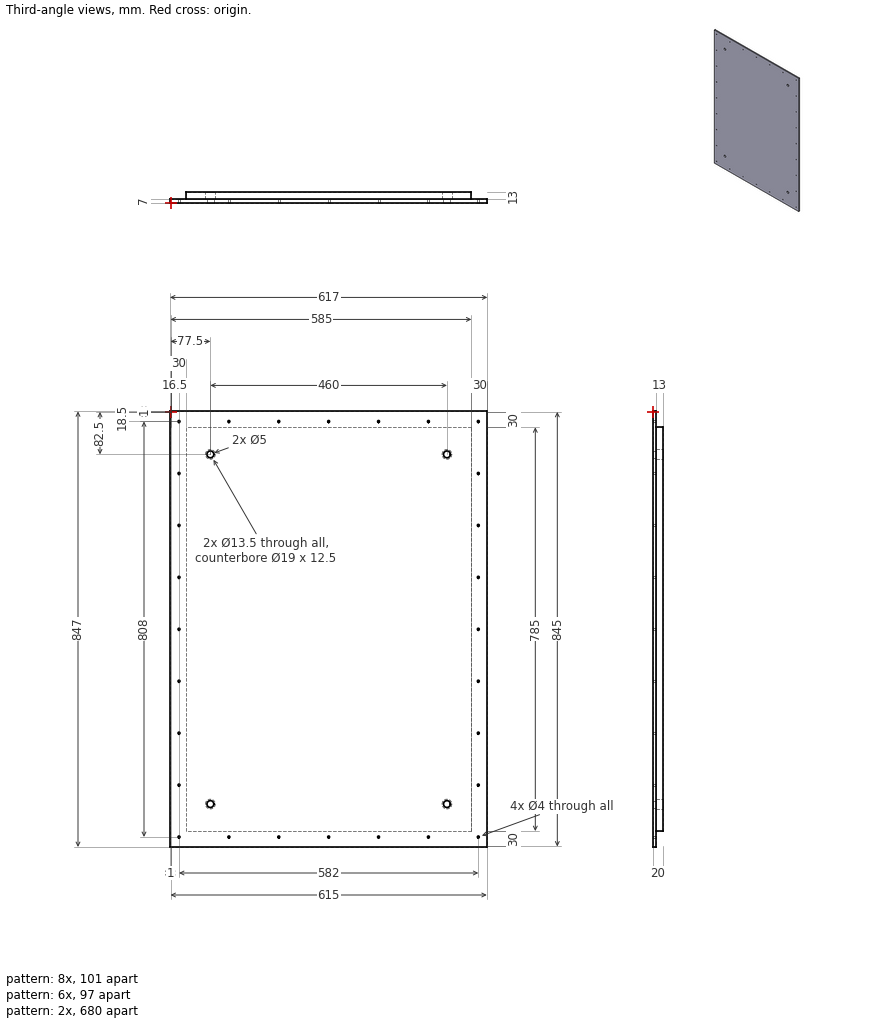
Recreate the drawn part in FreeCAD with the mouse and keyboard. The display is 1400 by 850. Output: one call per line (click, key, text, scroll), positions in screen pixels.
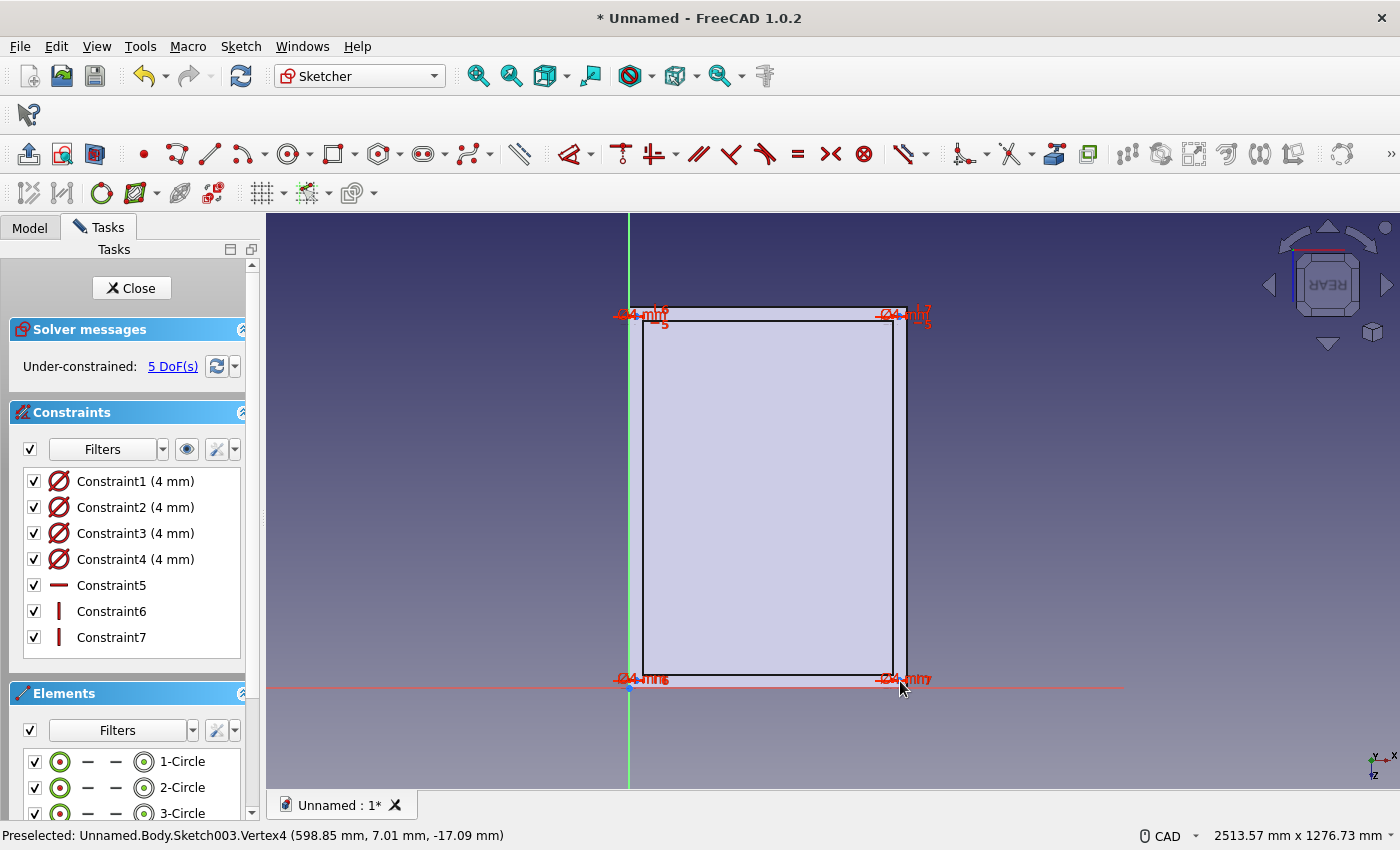
click(637, 681)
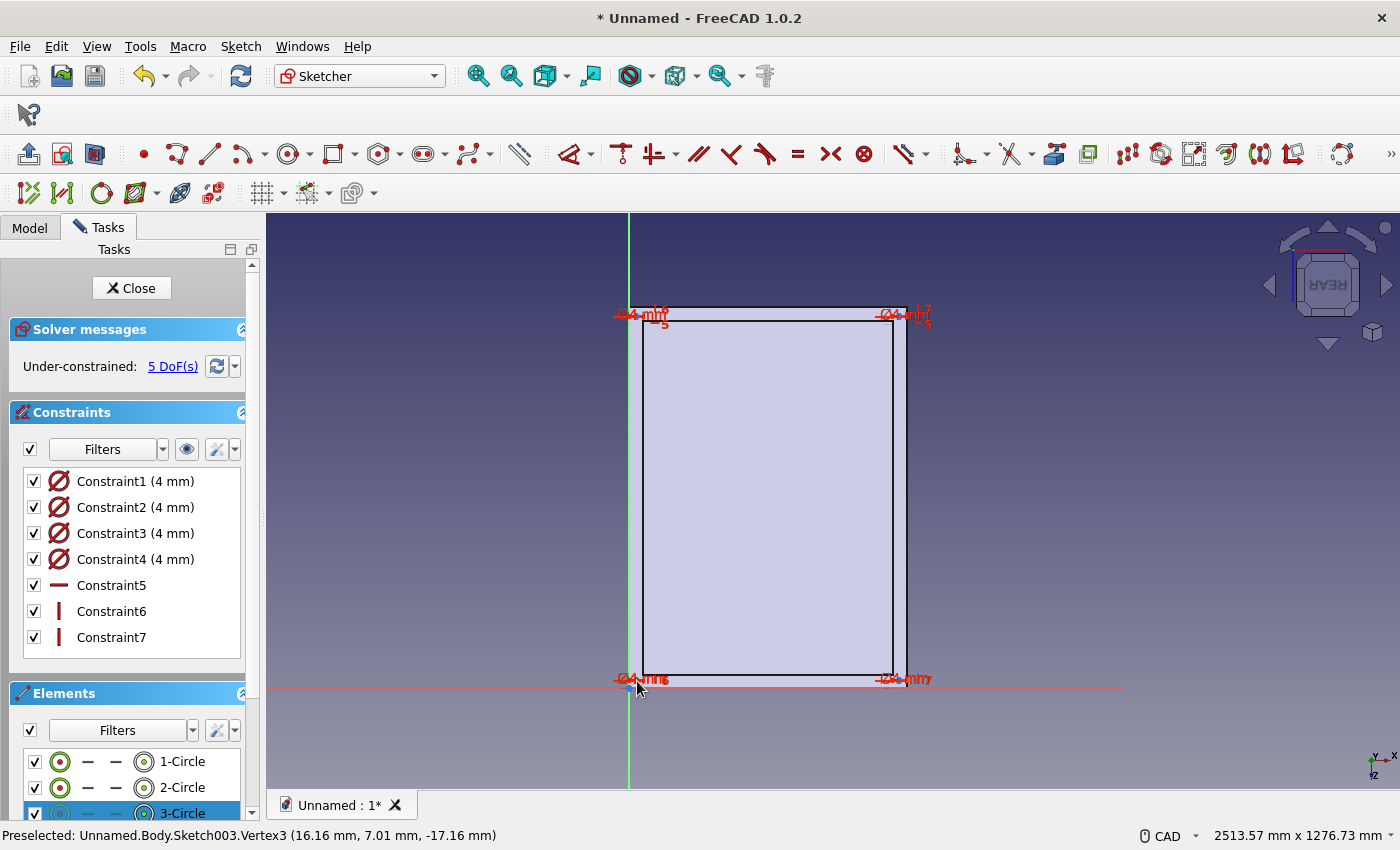
click(899, 681)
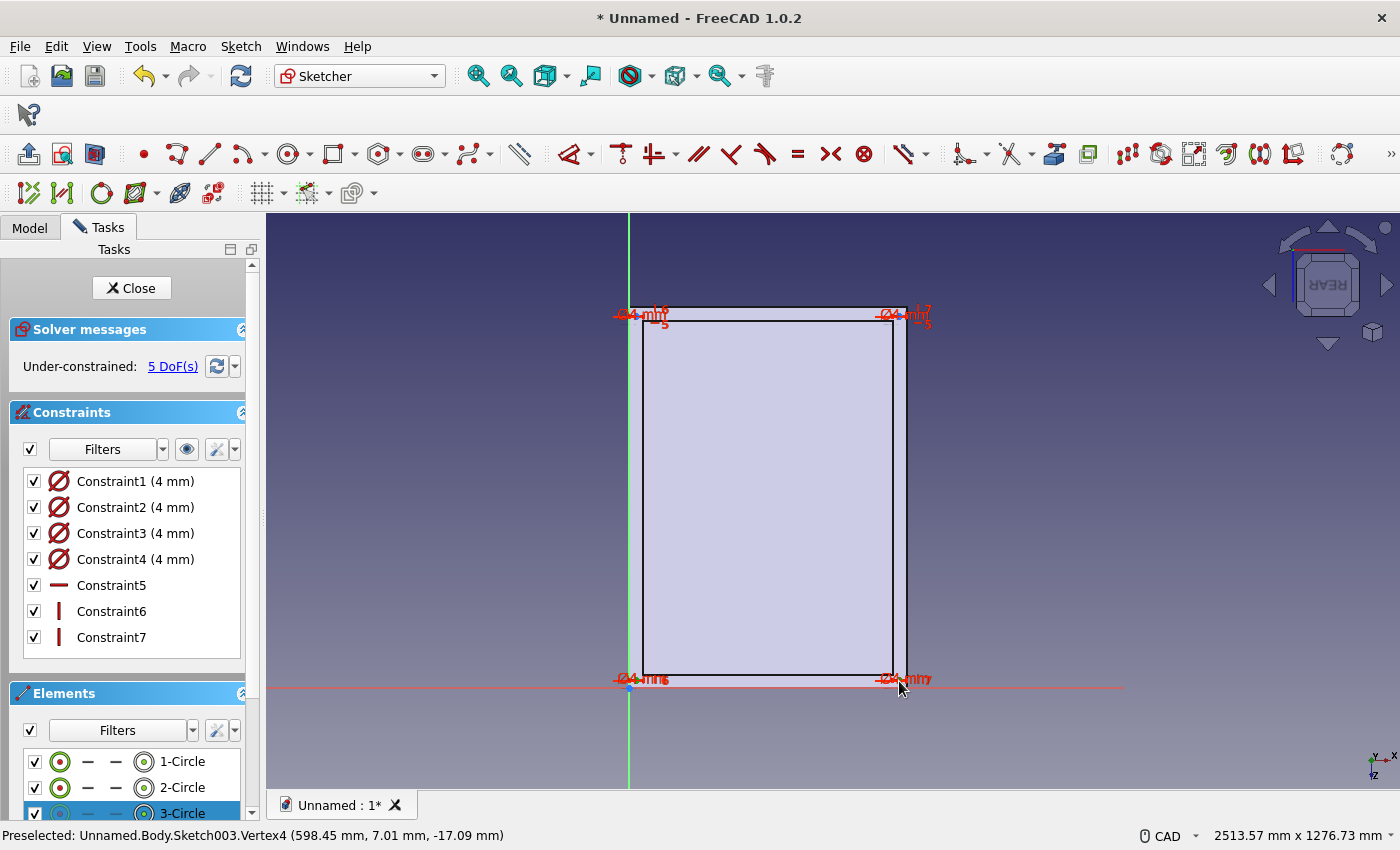
click(676, 154)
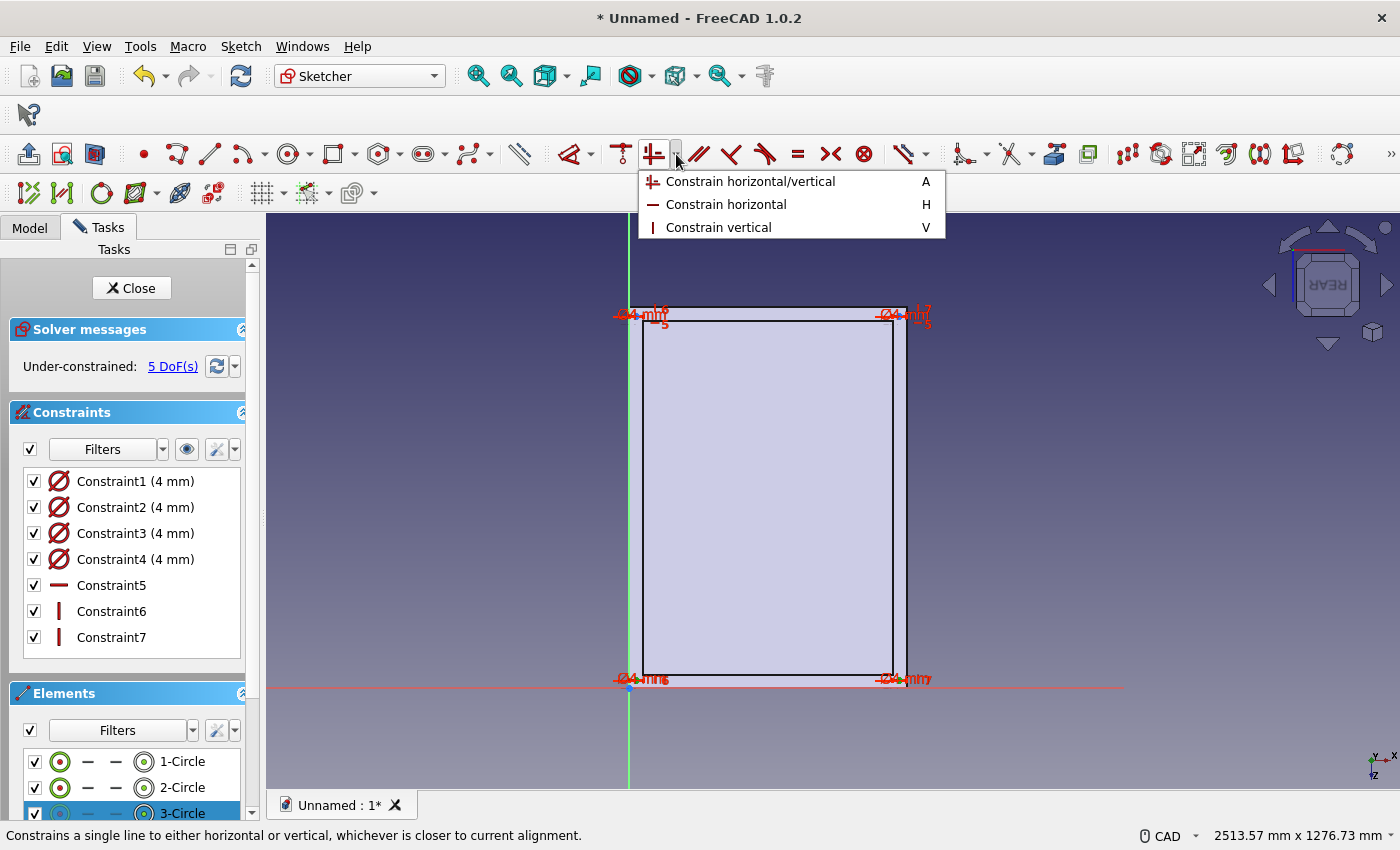
click(792, 204)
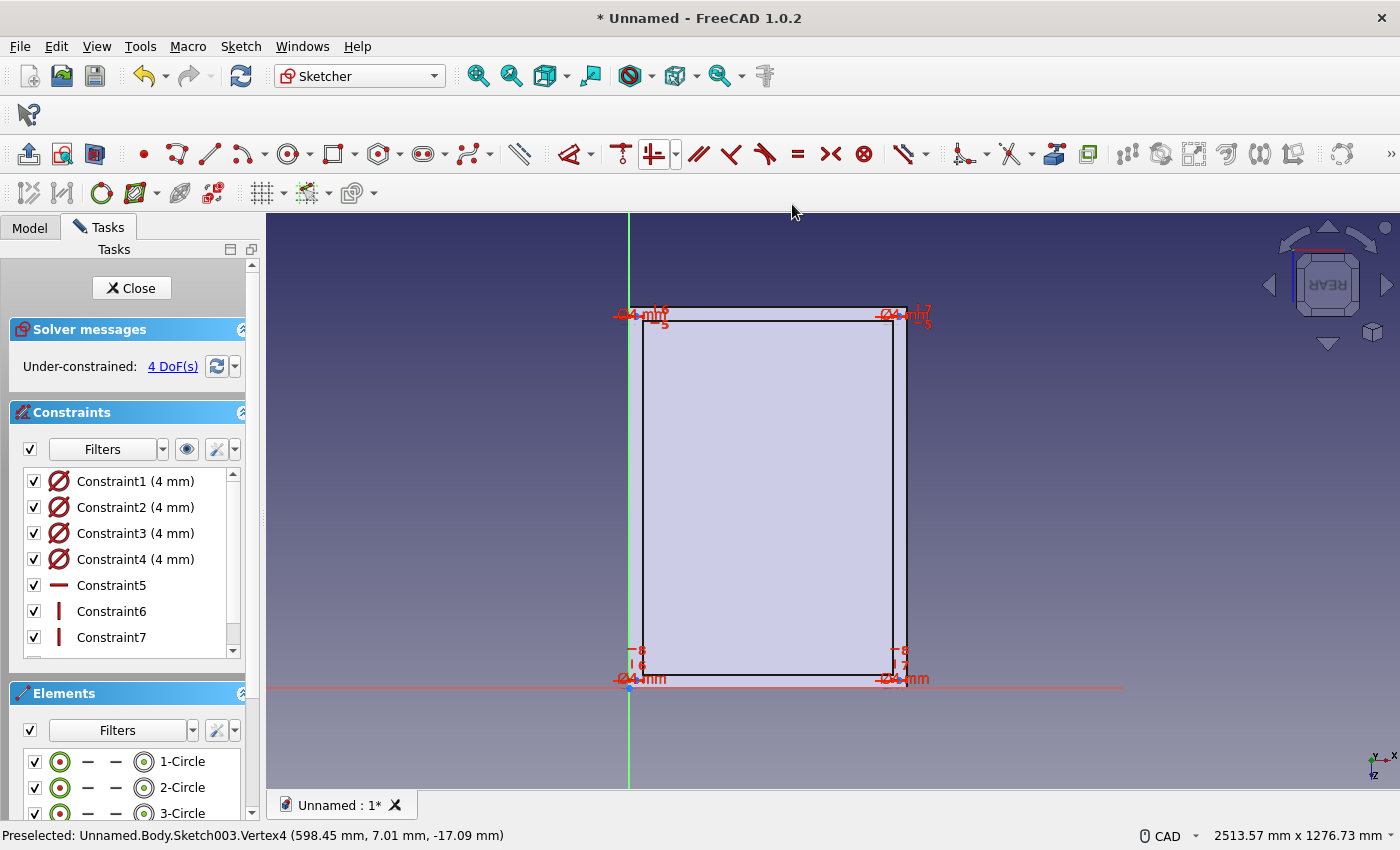
click(568, 154)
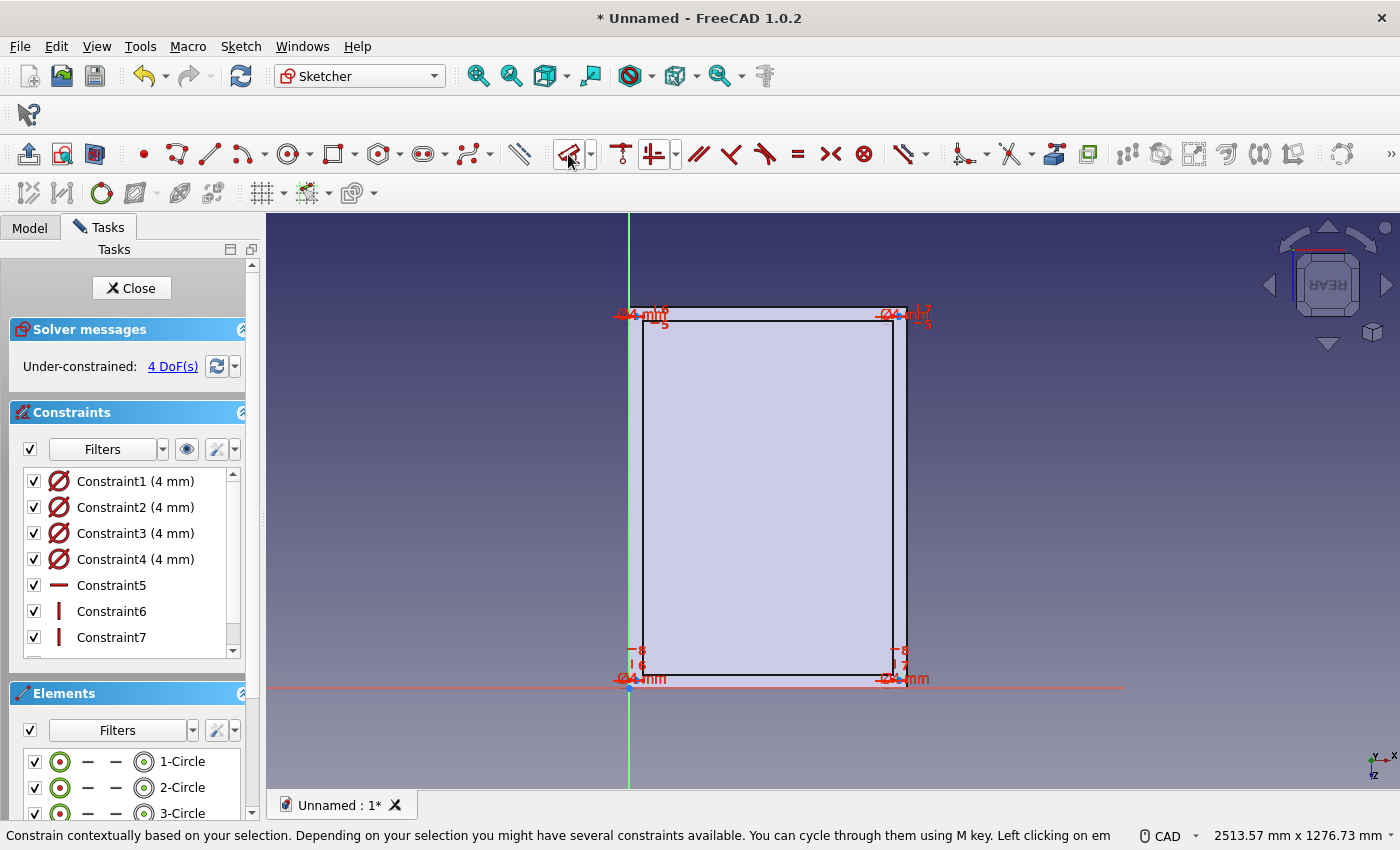
scroll(637, 317, up, 9)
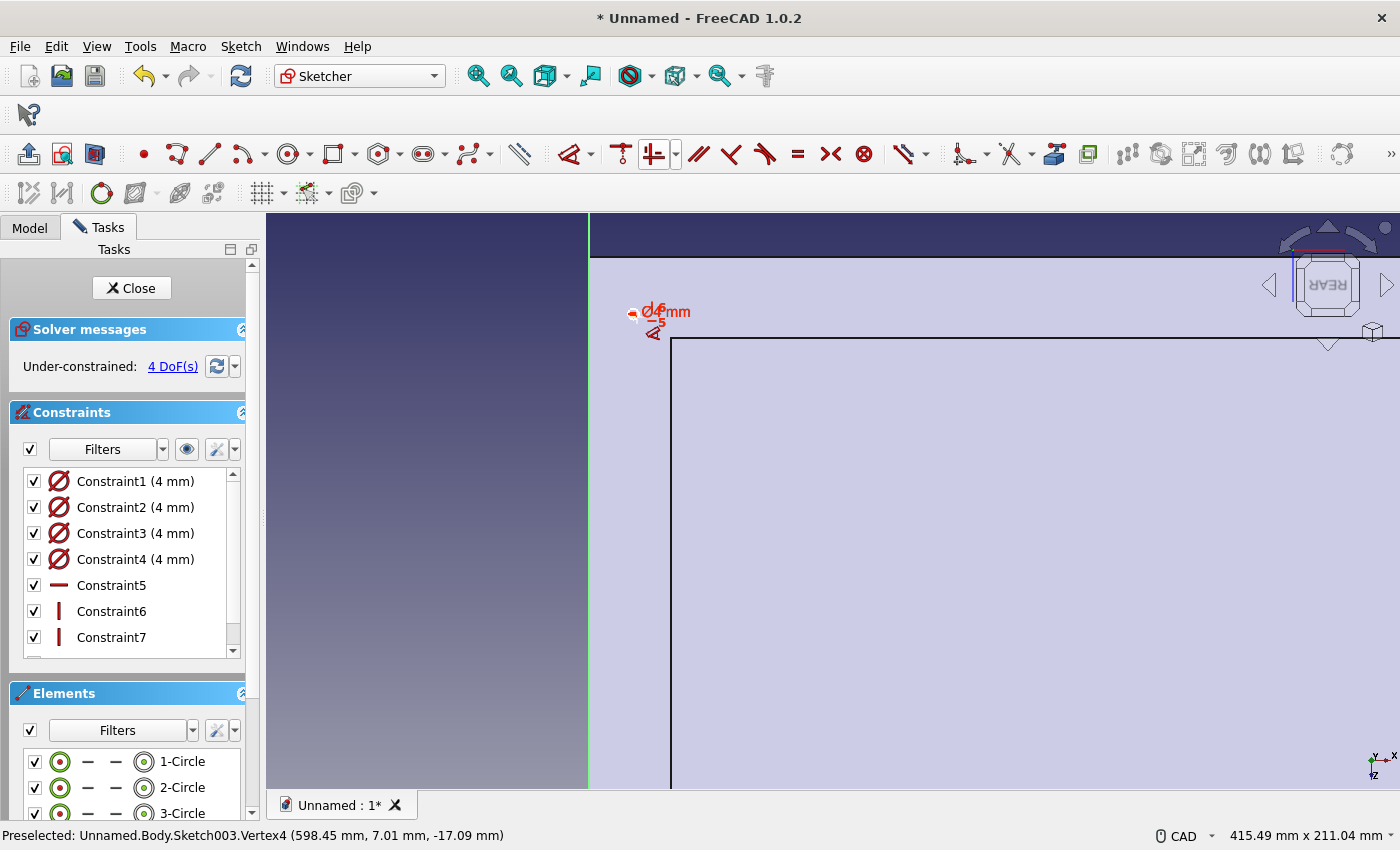
click(633, 314)
click(611, 280)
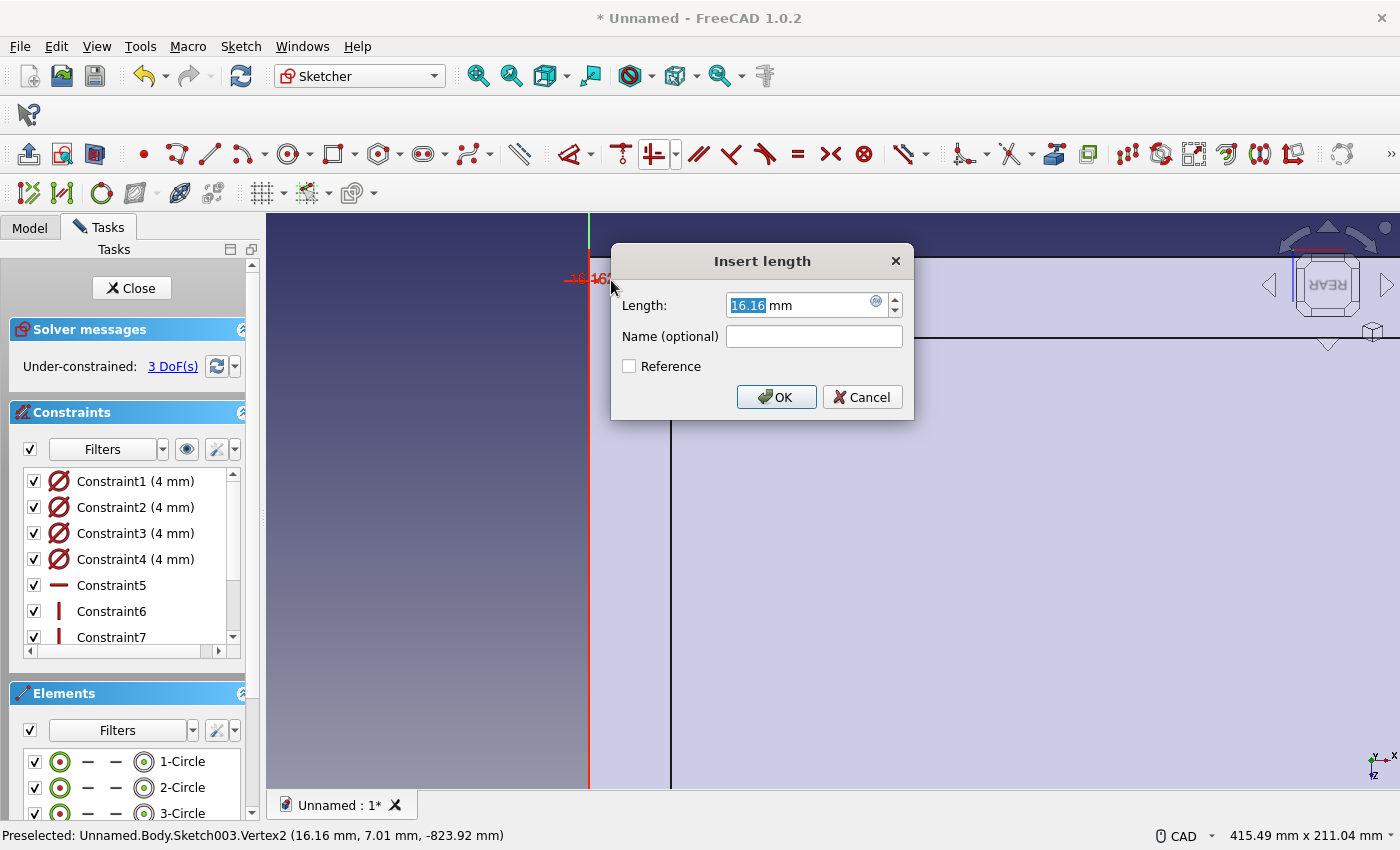
text(16.5)
key(Return)